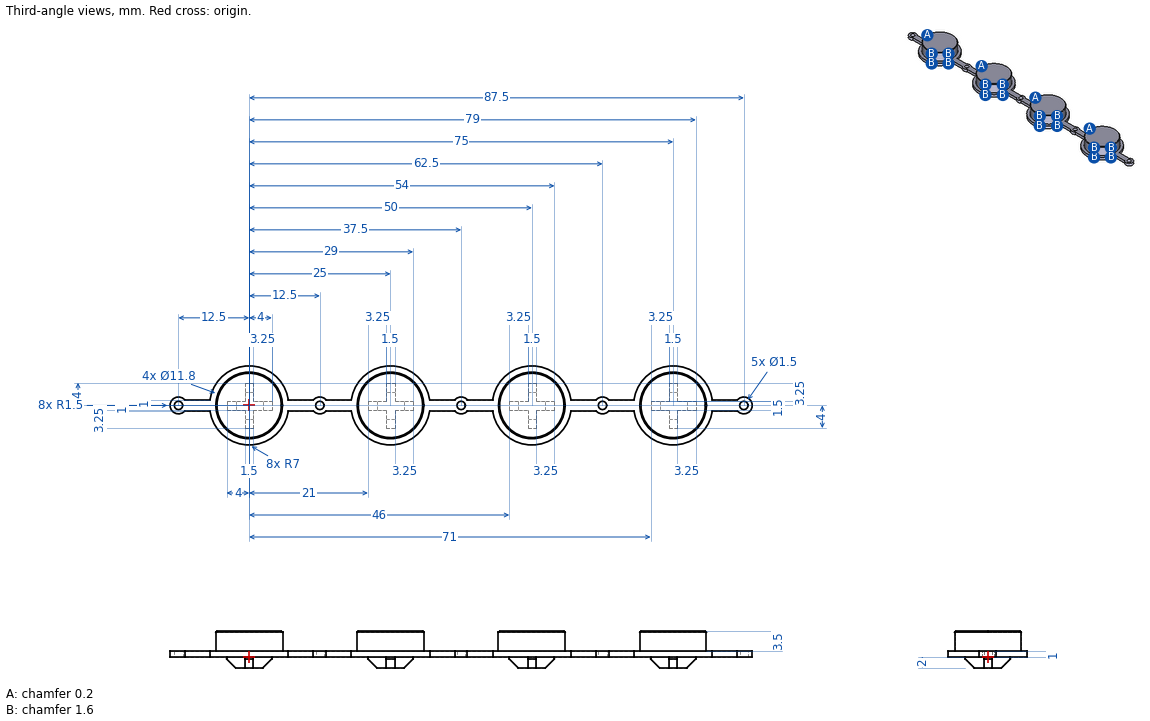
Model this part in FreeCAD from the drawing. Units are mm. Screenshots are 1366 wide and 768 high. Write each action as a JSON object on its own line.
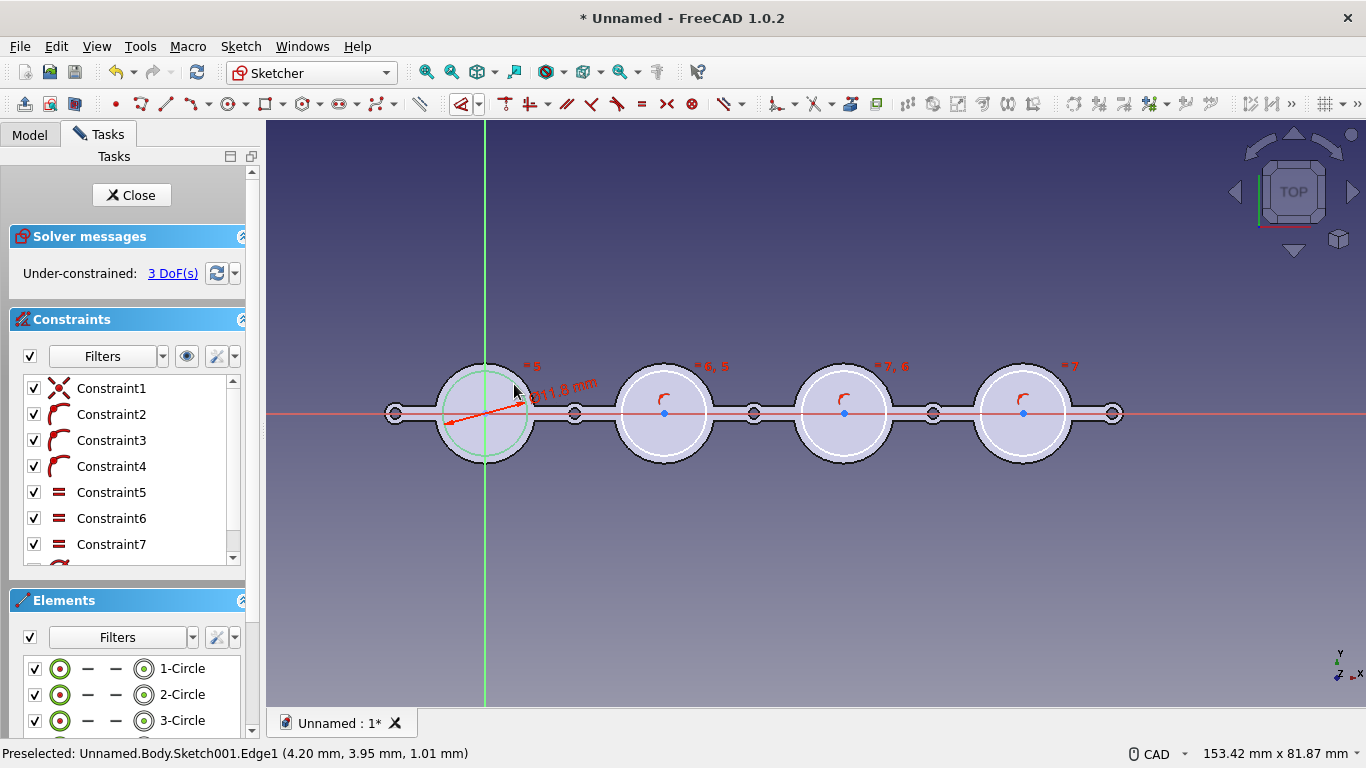
{"action": "left_click", "coordinate": [664, 414]}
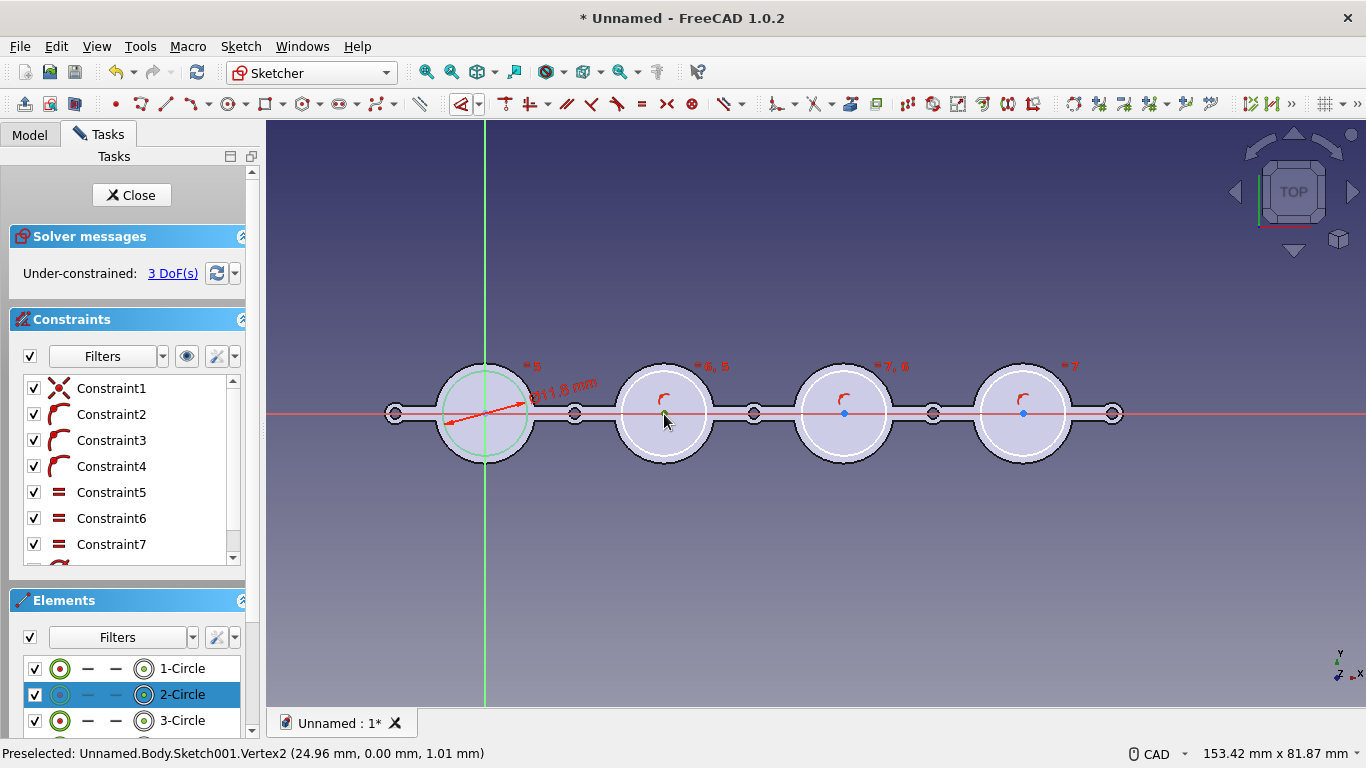
{"action": "key", "text": "l"}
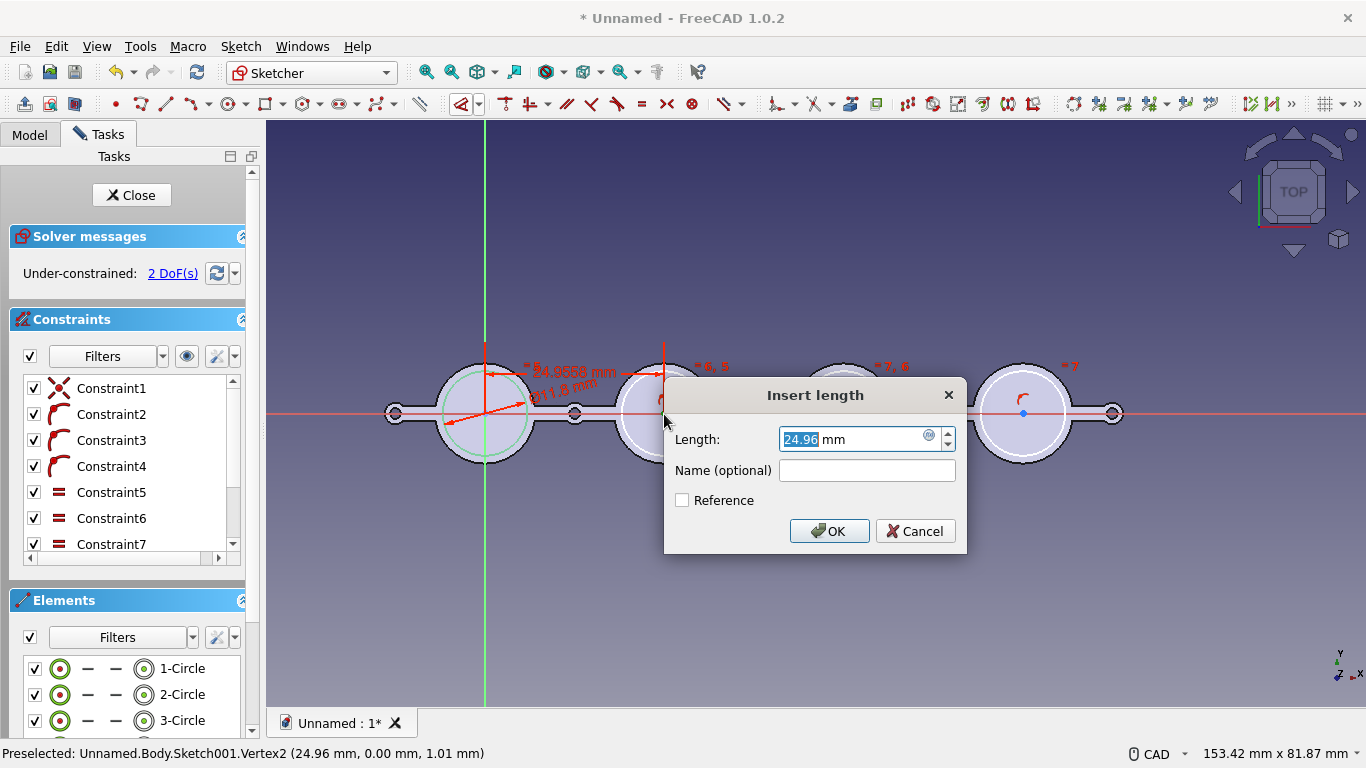
{"action": "type", "text": "25"}
{"action": "key", "text": "Return"}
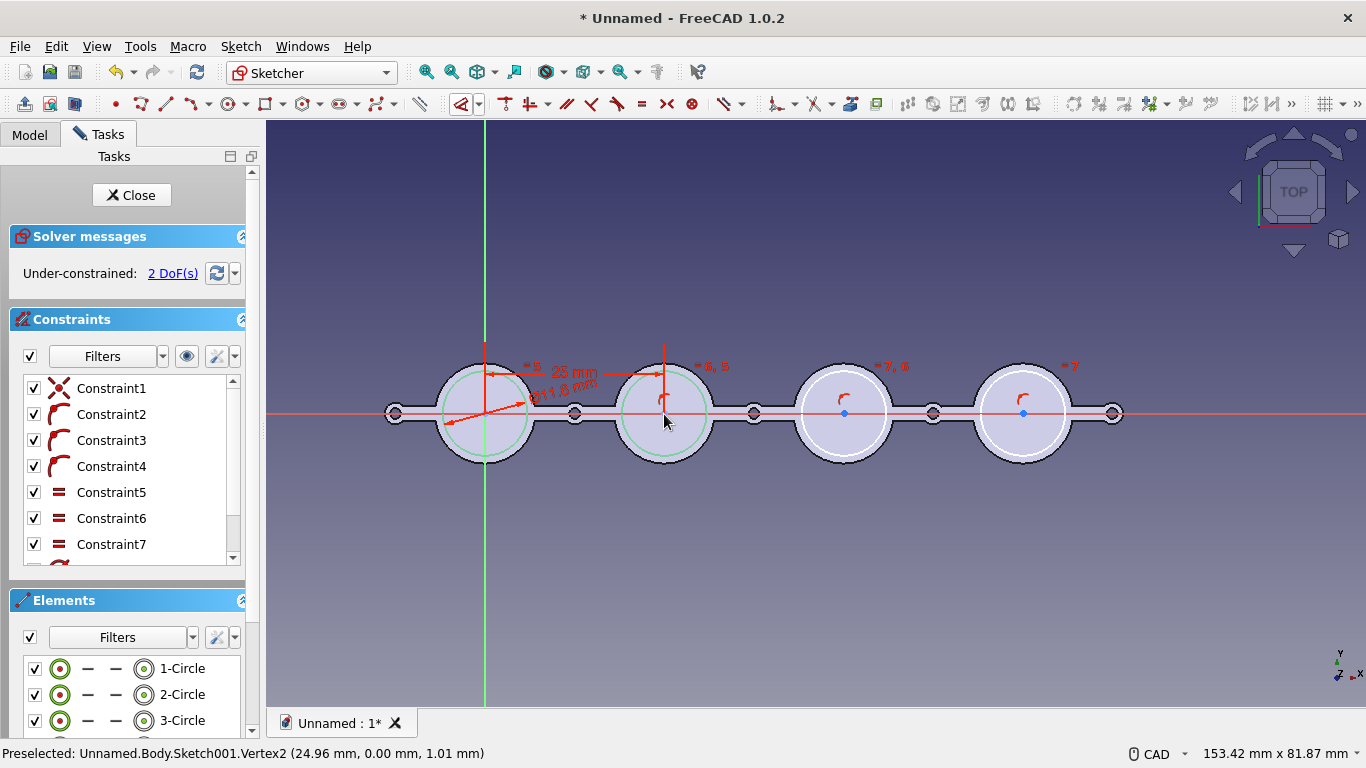
{"action": "left_click", "coordinate": [844, 414]}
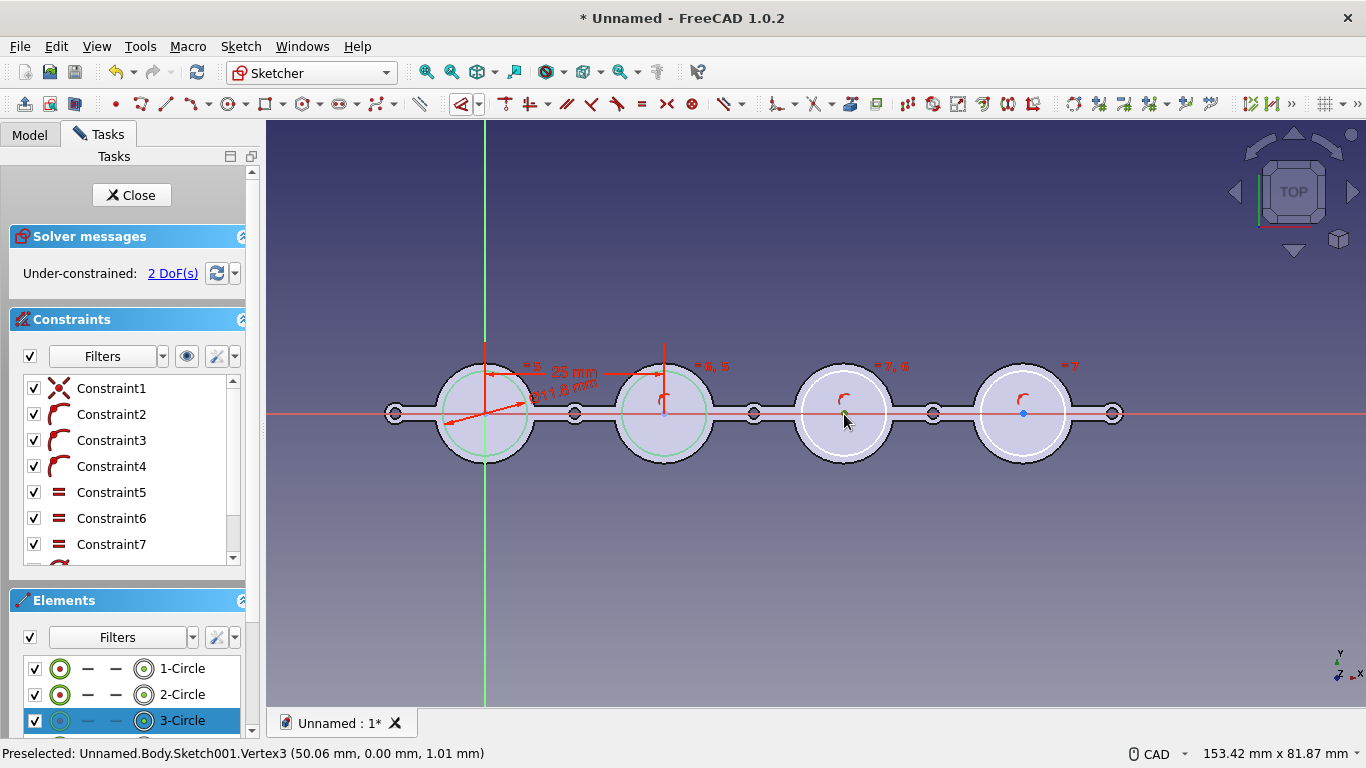
{"action": "key", "text": "l"}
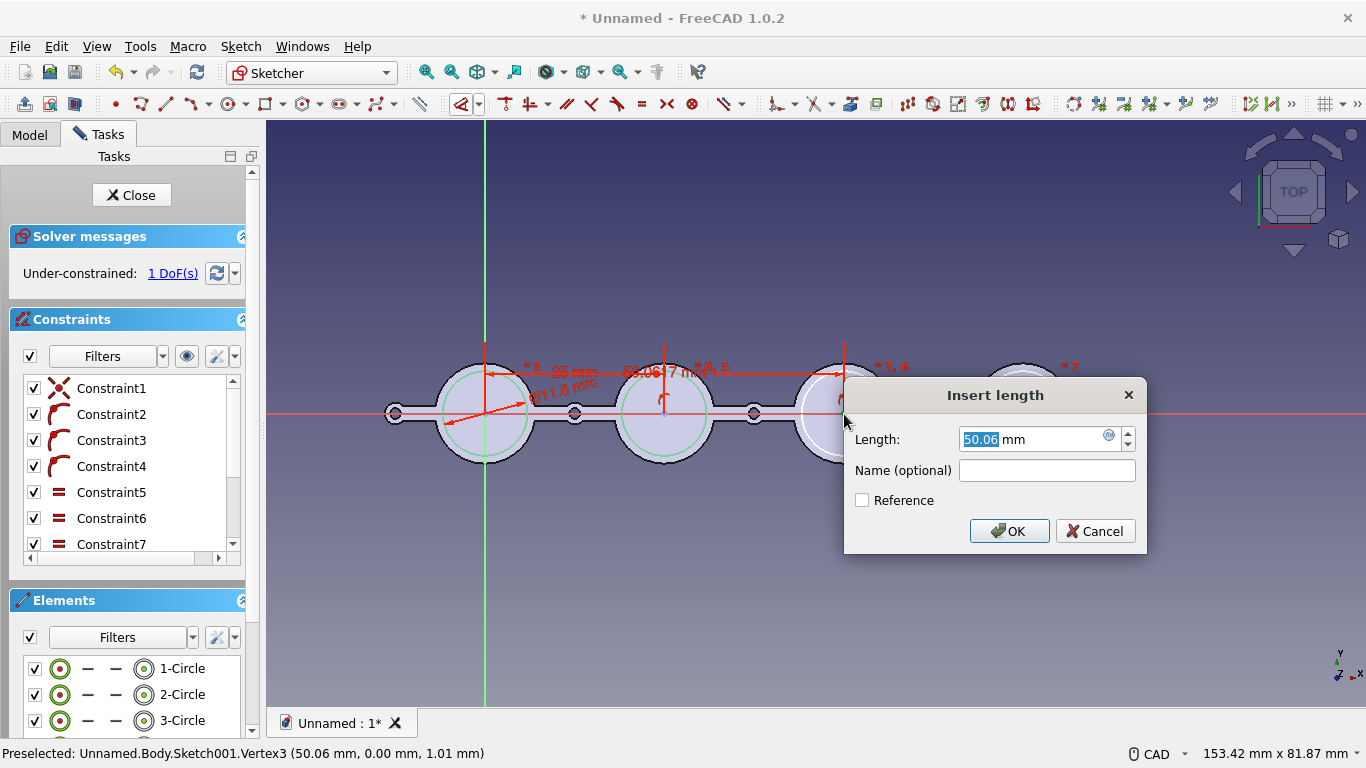
{"action": "type", "text": "50"}
{"action": "key", "text": "Return"}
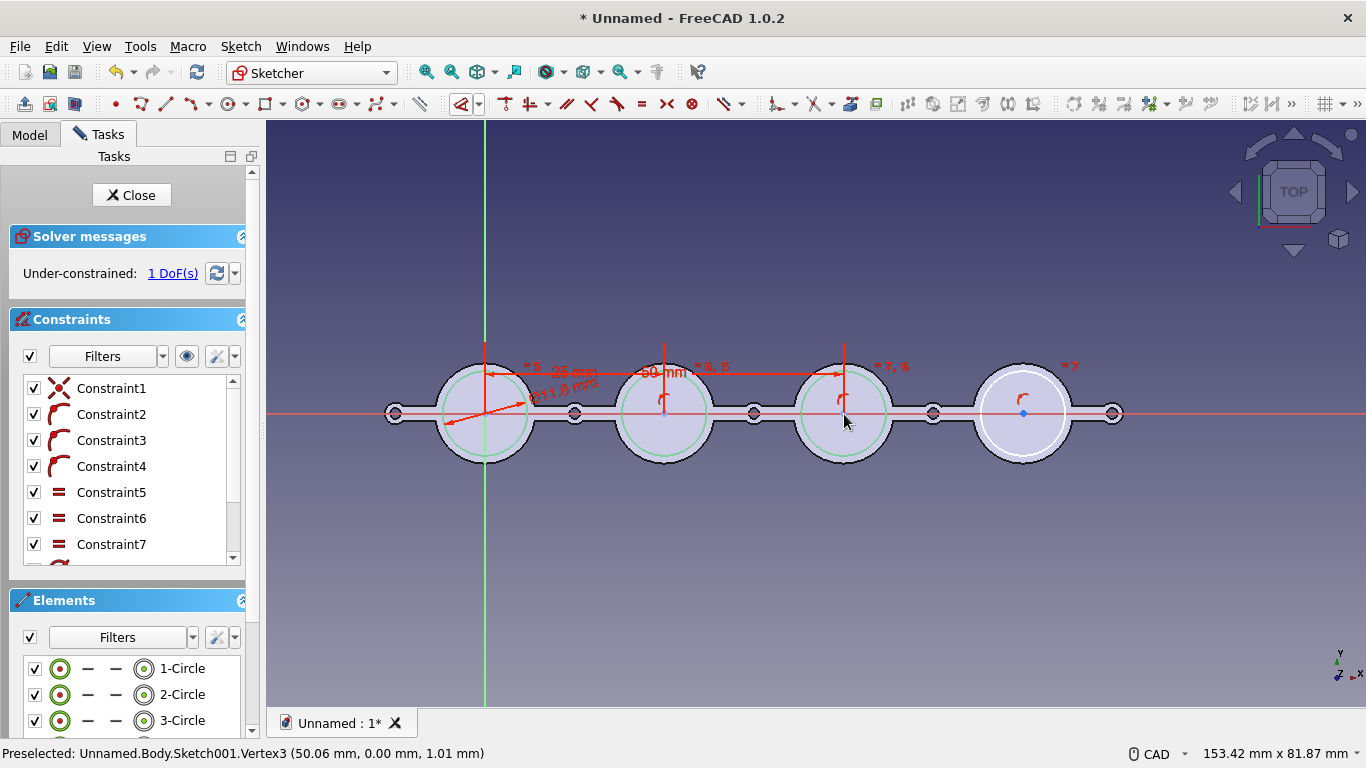
{"action": "left_click", "coordinate": [1023, 414]}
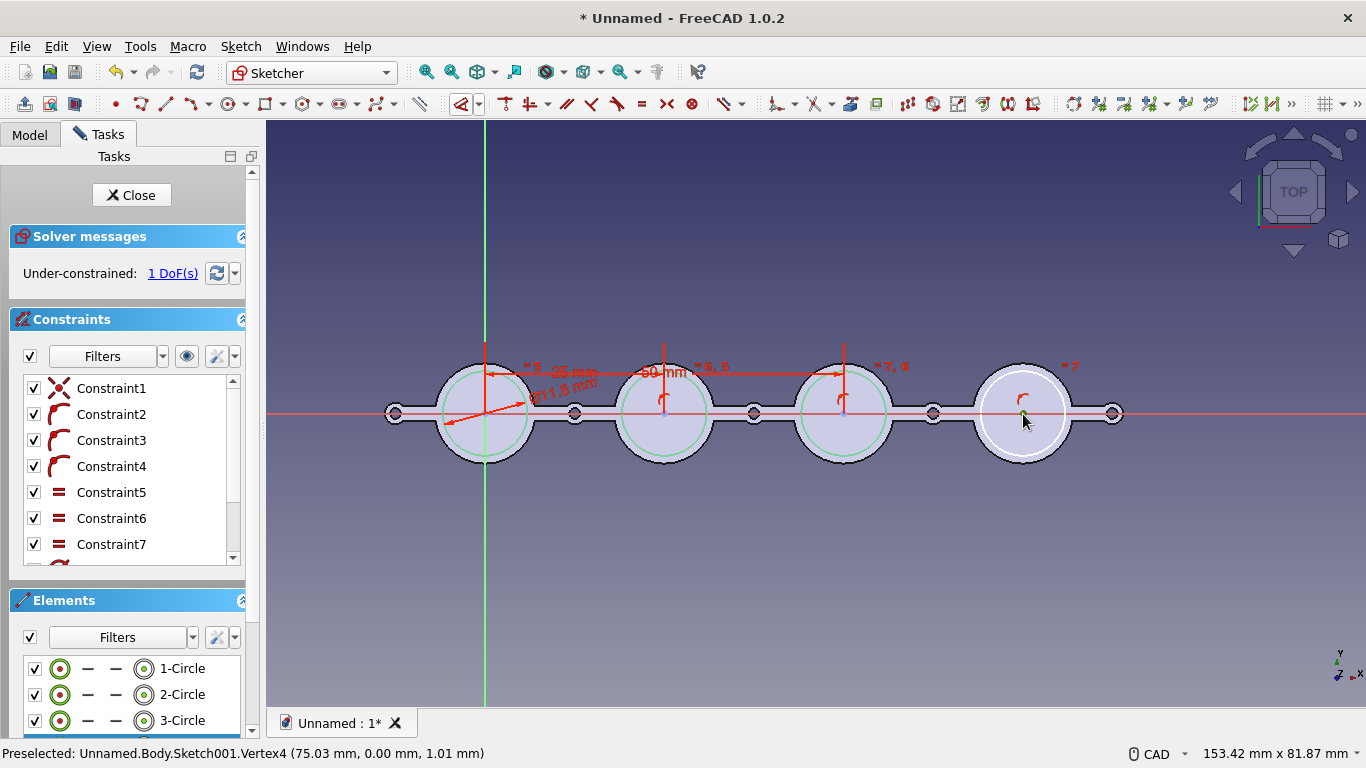
{"action": "key", "text": "l"}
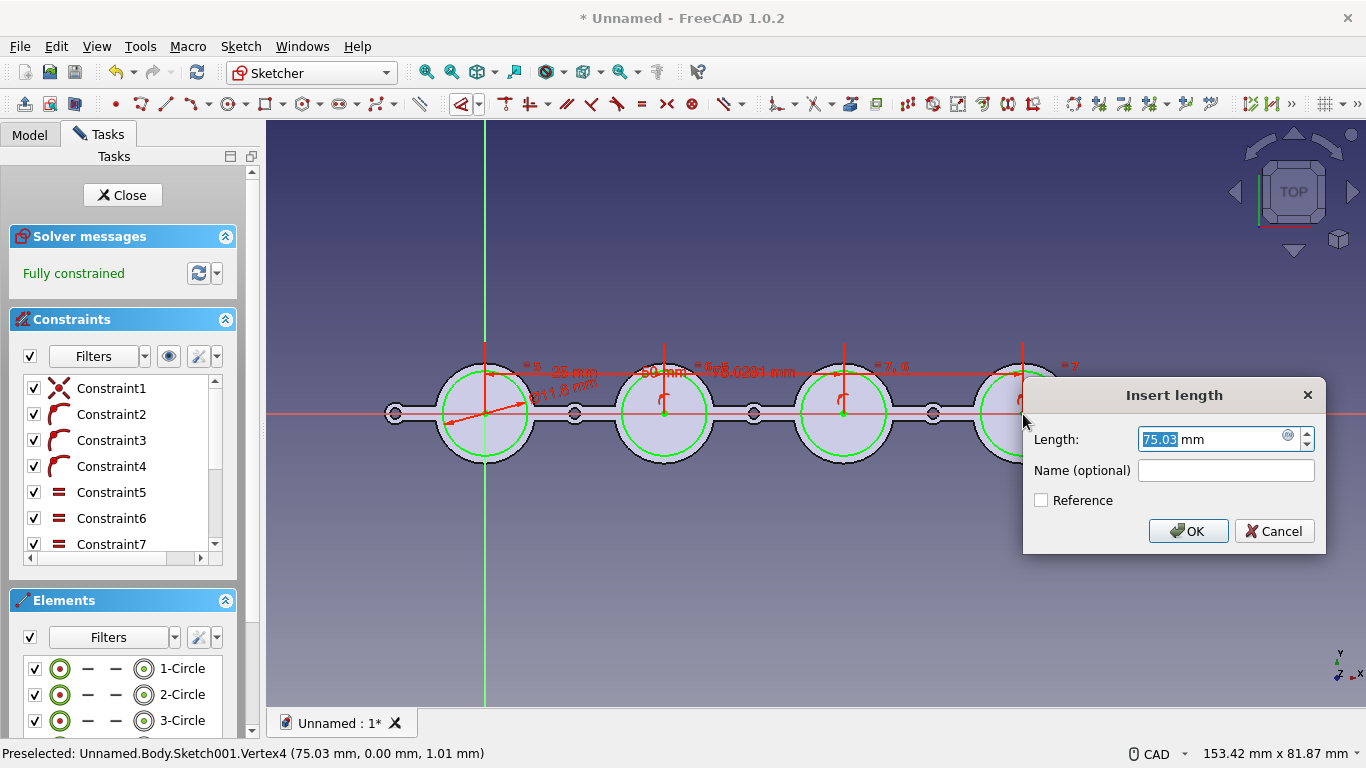
{"action": "type", "text": "75"}
{"action": "key", "text": "Return"}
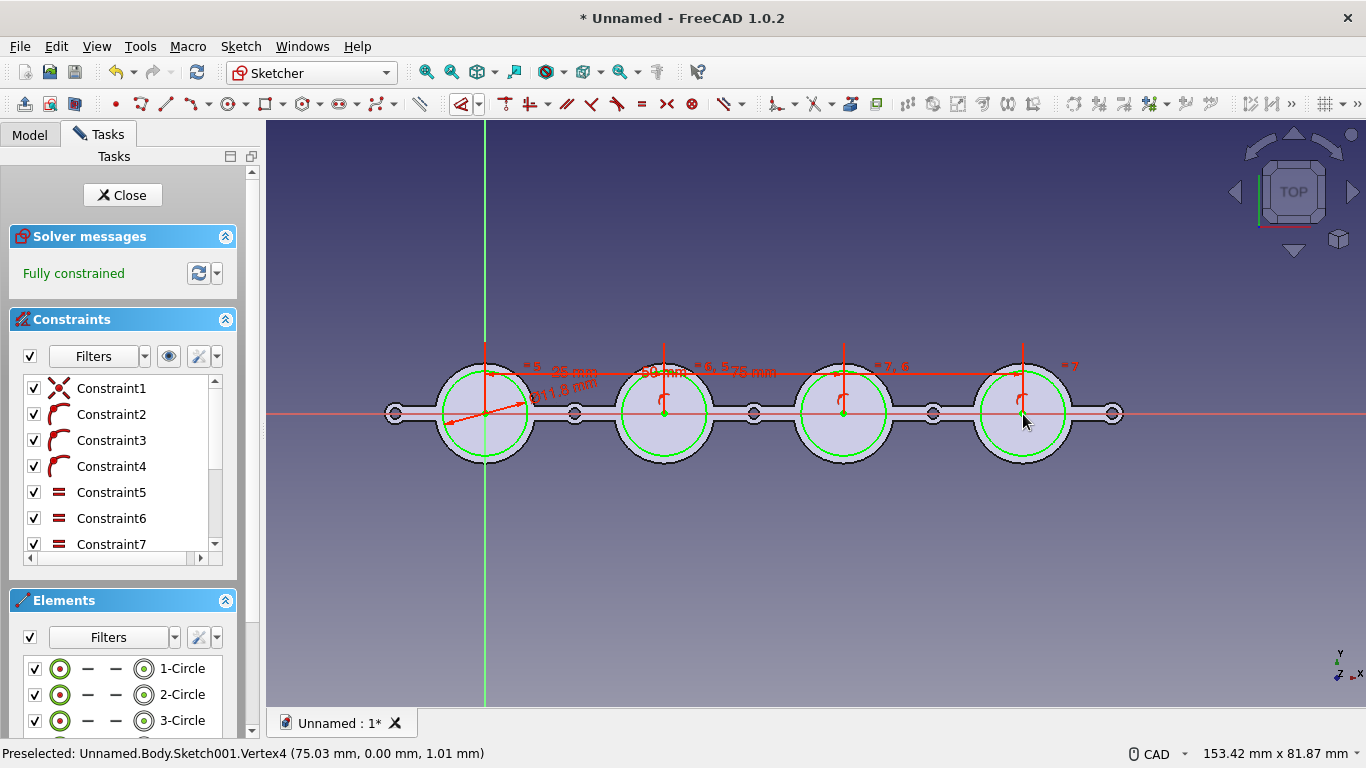
{"action": "left_click", "coordinate": [123, 195]}